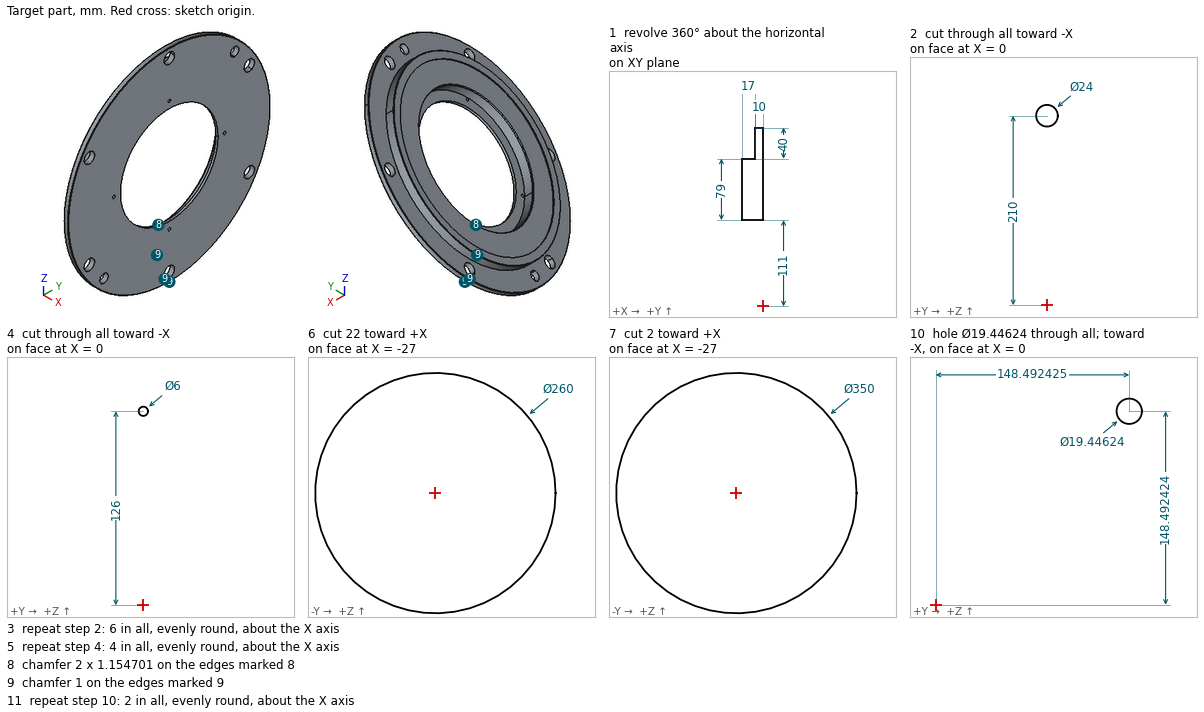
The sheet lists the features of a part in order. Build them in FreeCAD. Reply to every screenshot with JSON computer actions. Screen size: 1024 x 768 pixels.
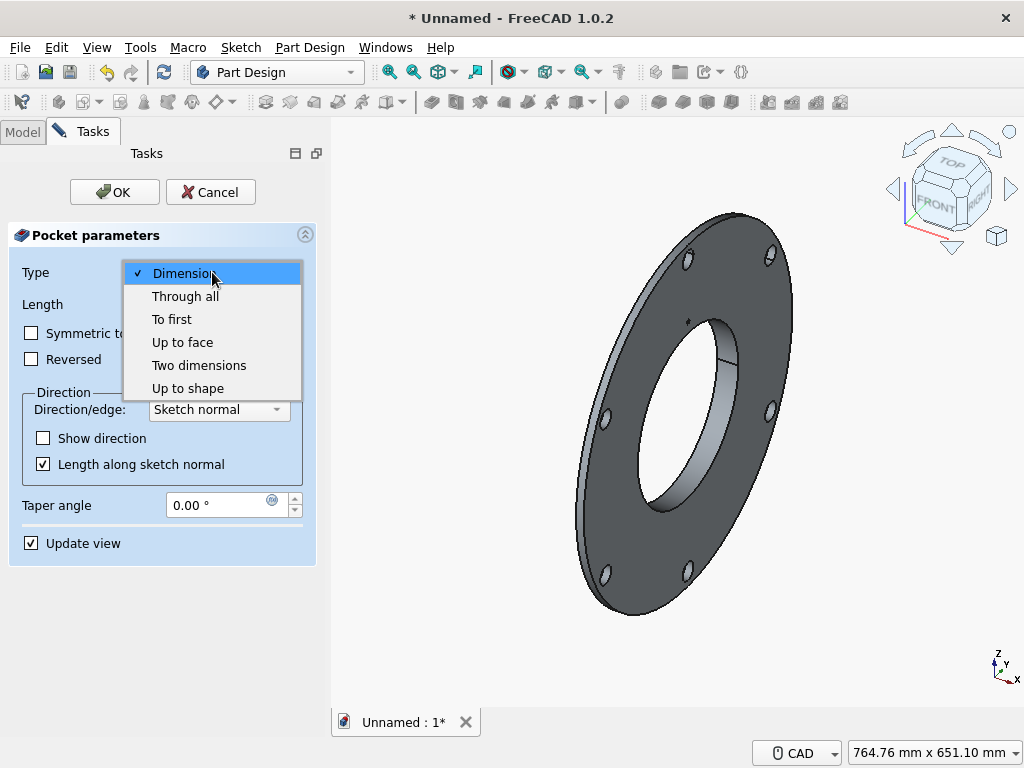
{"action": "left_click", "coordinate": [212, 296]}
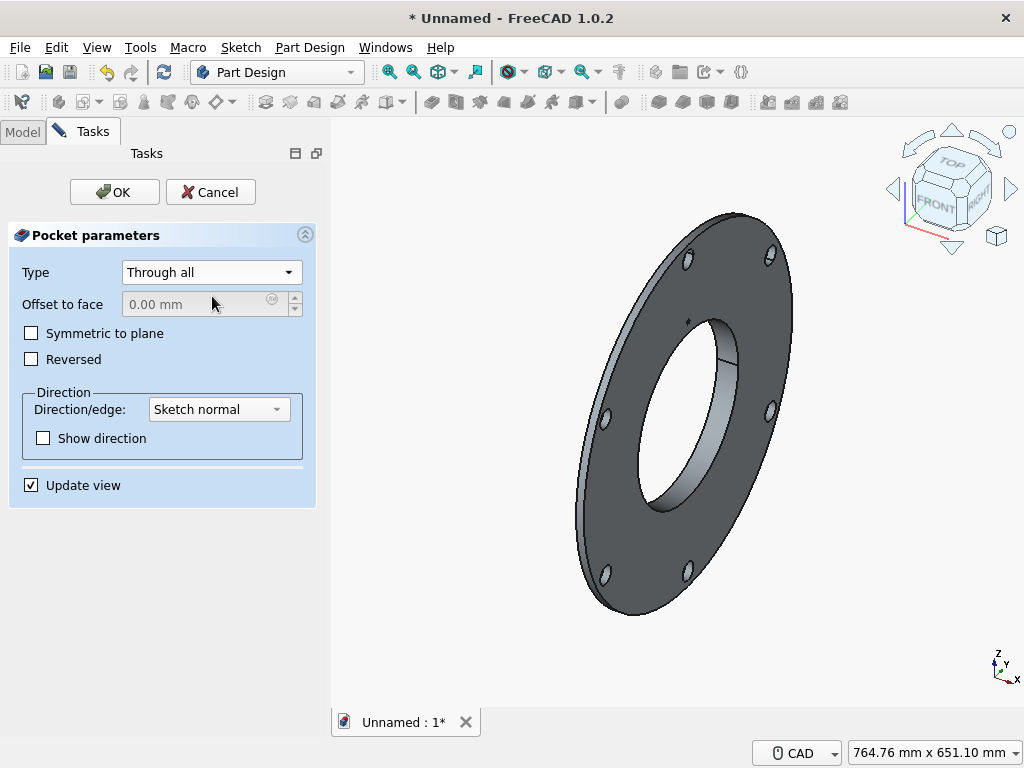
{"action": "left_click", "coordinate": [115, 192]}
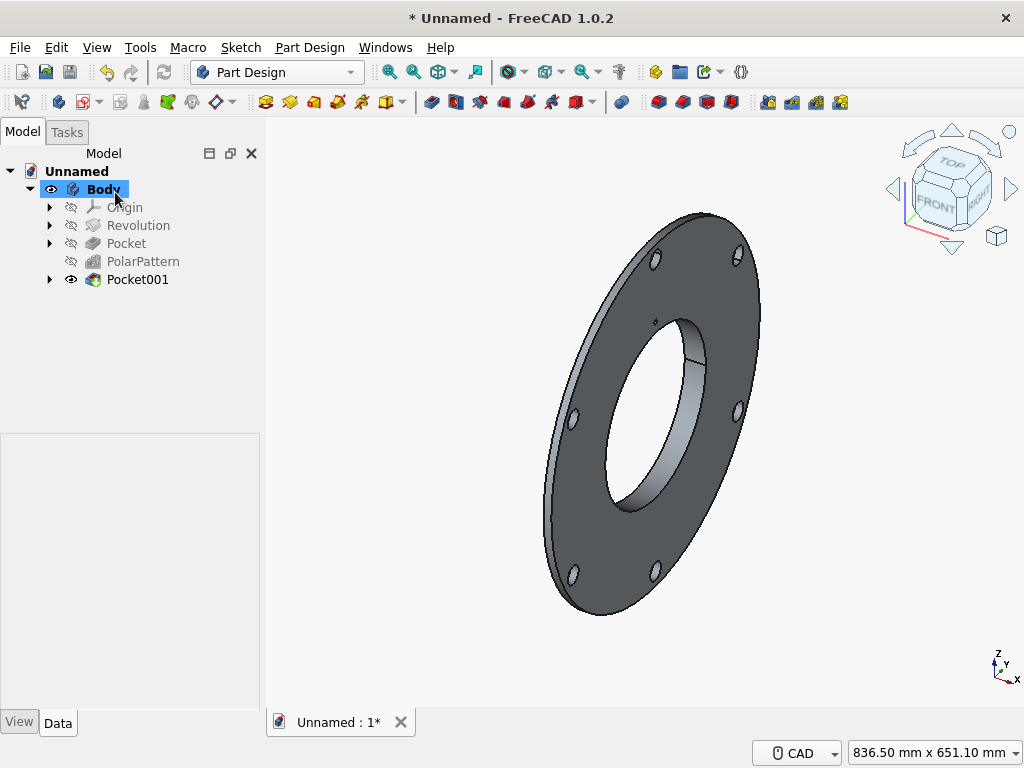
{"action": "left_click", "coordinate": [116, 279]}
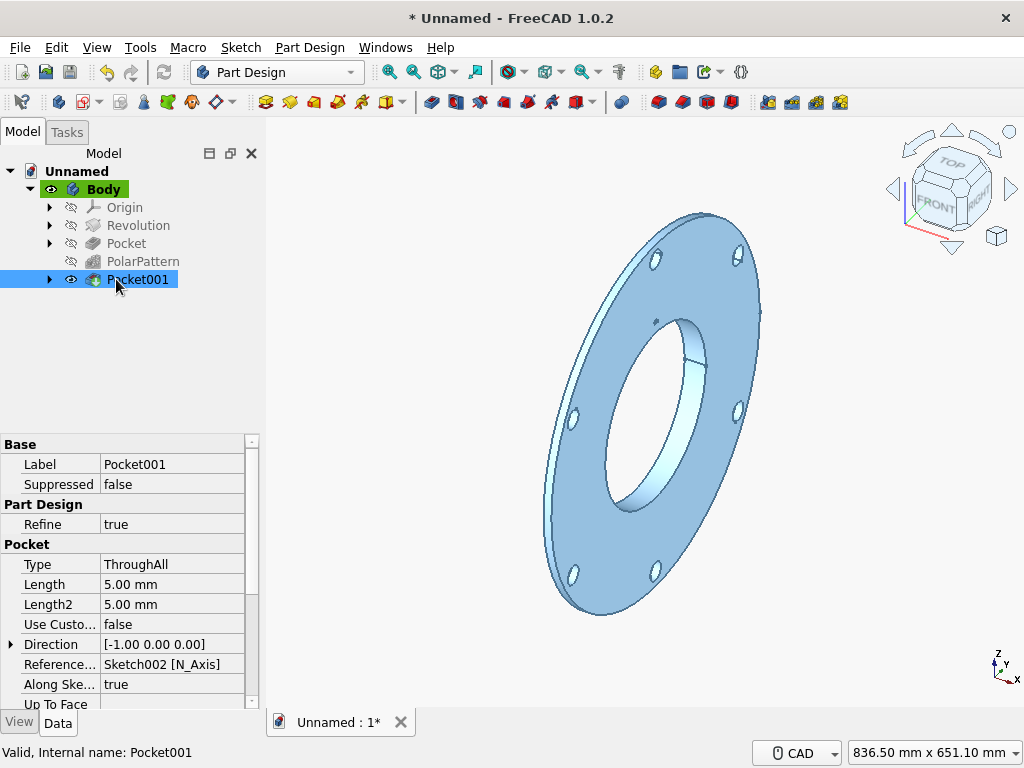
{"action": "left_click", "coordinate": [816, 102]}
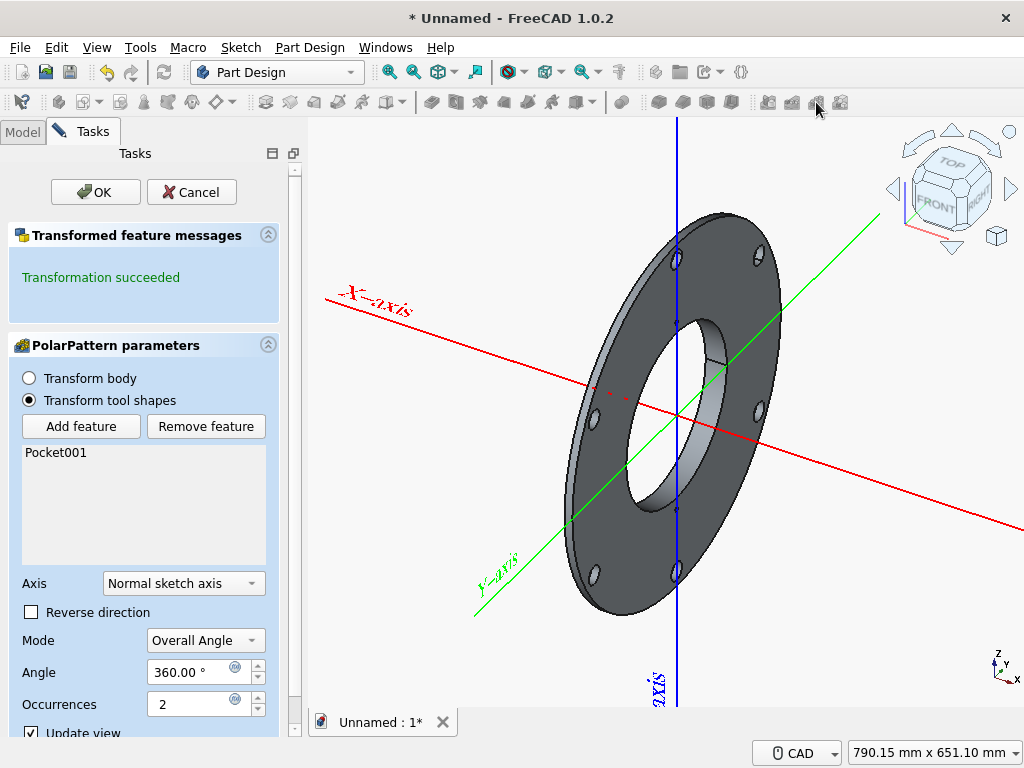
{"action": "left_click", "coordinate": [184, 584]}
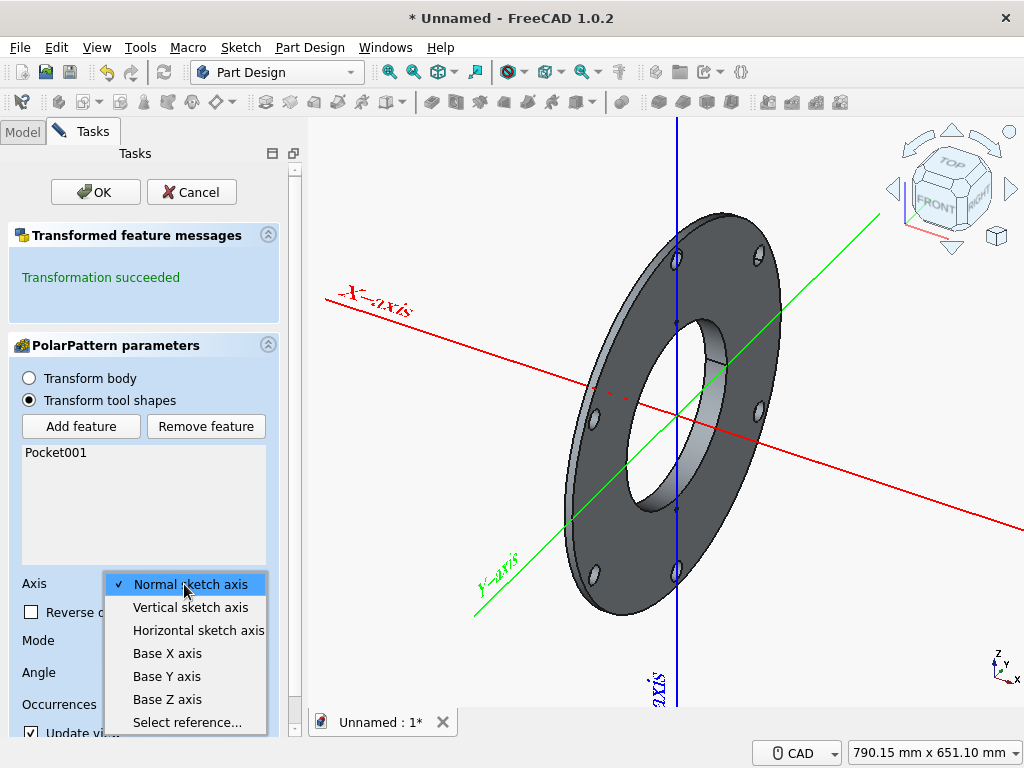
{"action": "left_click", "coordinate": [184, 654]}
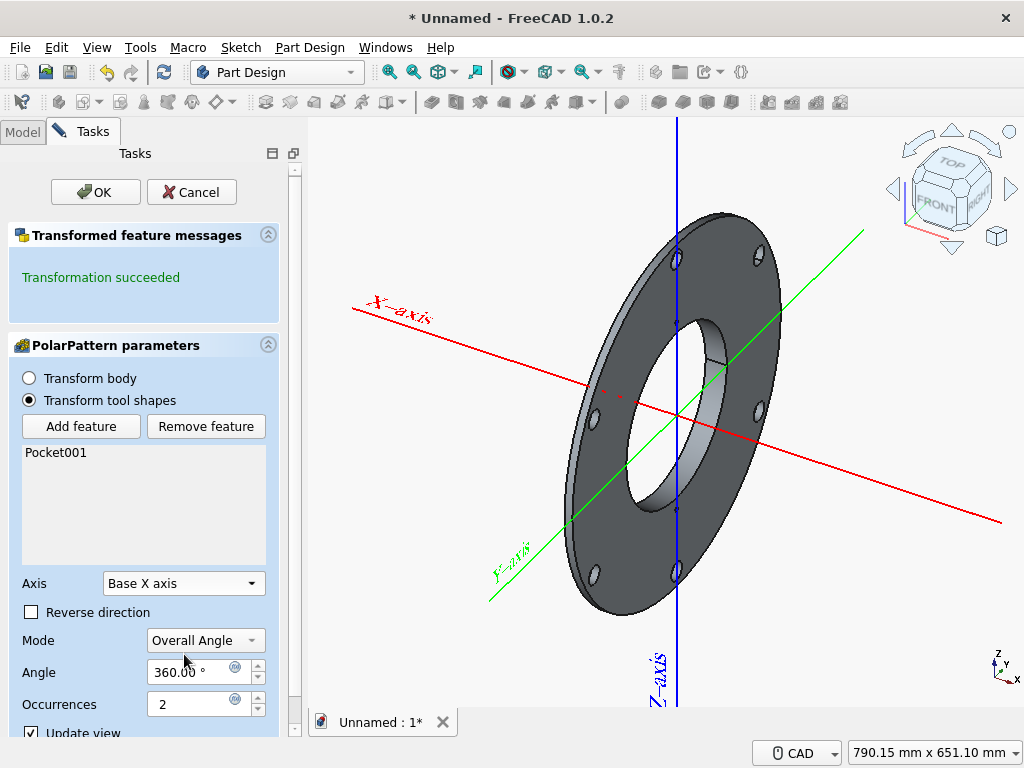
{"action": "triple_click", "coordinate": [198, 704]}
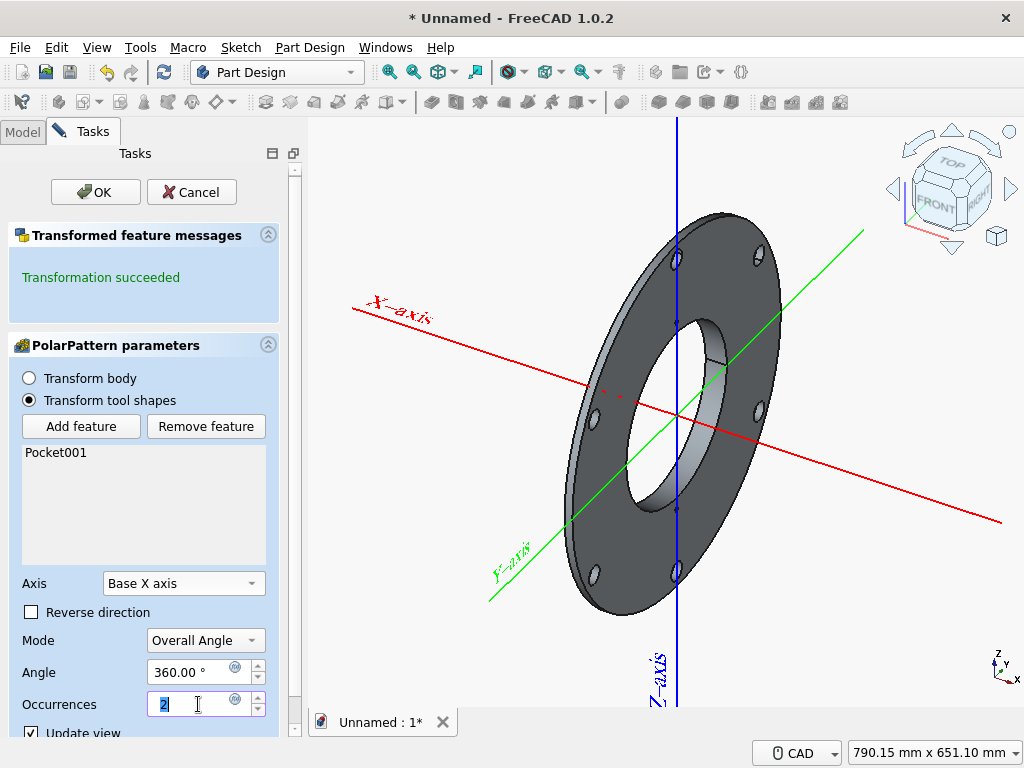
{"action": "type", "text": "4"}
{"action": "key", "text": "Tab"}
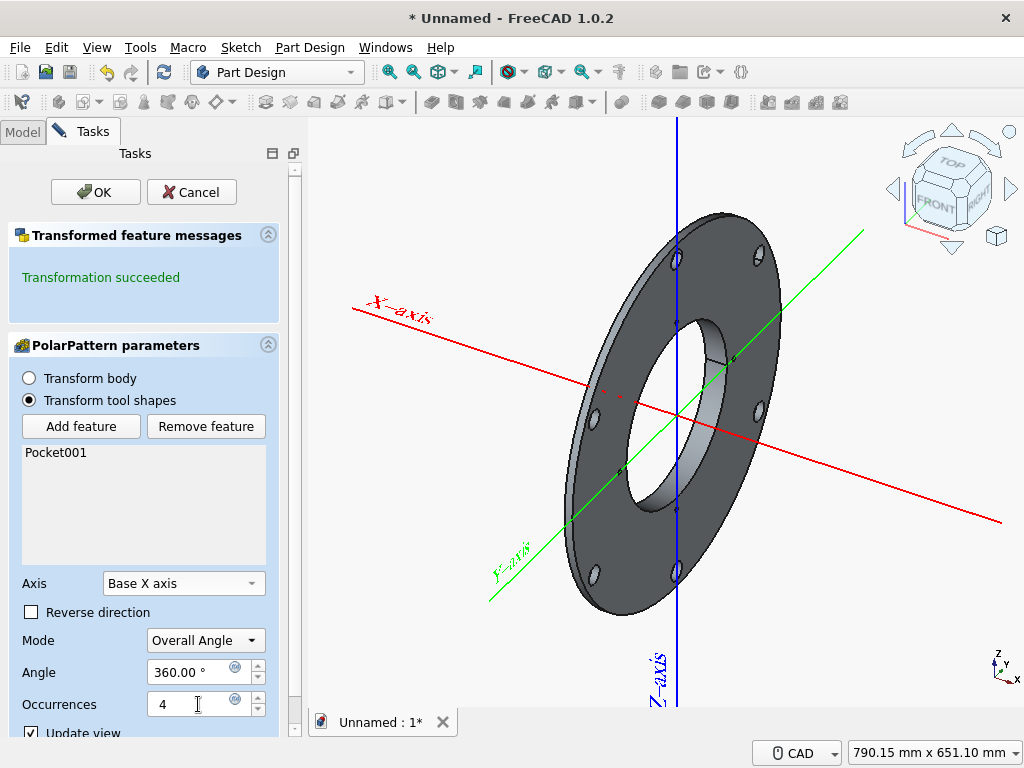
{"action": "left_click", "coordinate": [96, 192]}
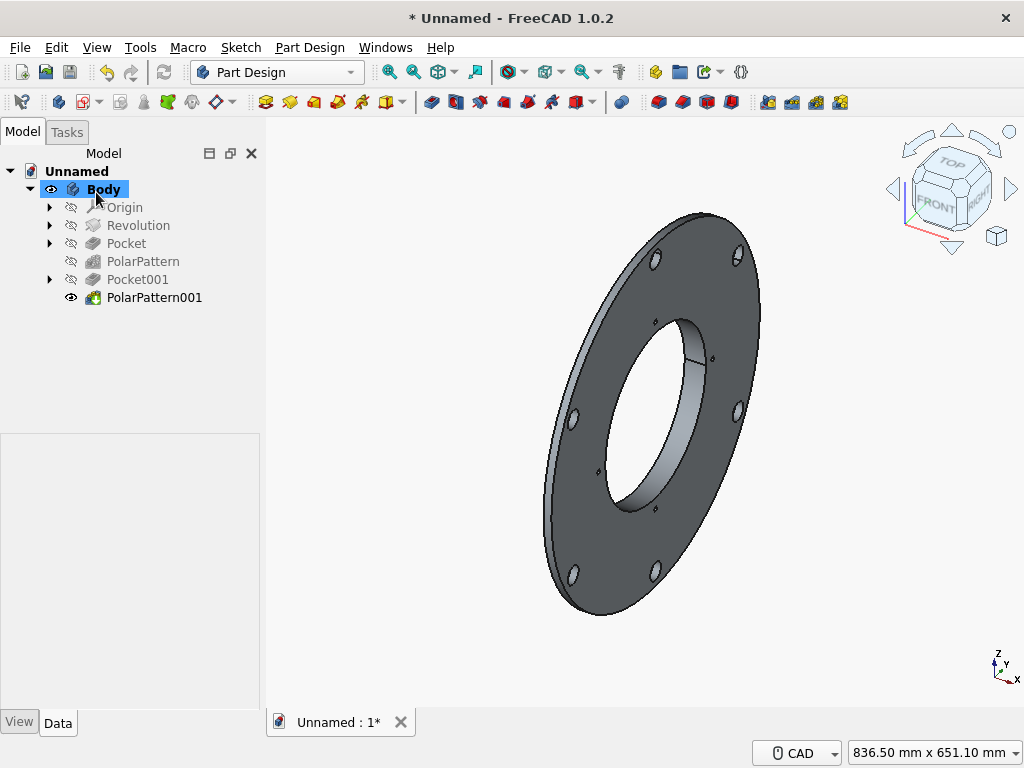
{"action": "key", "text": "6"}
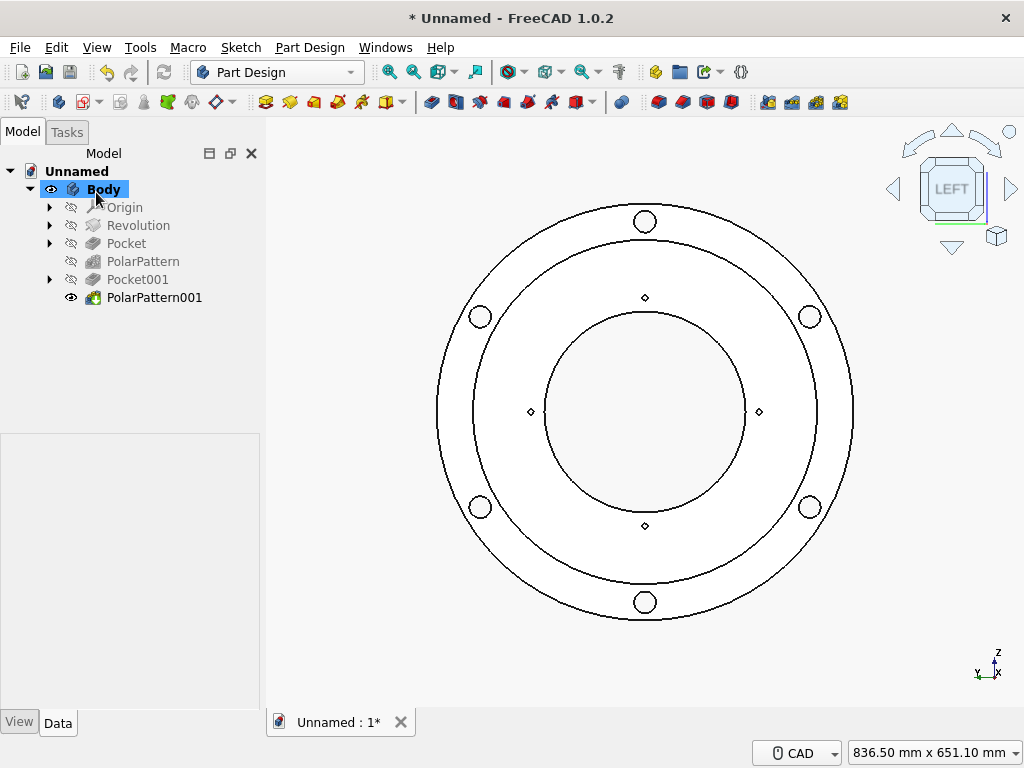
{"action": "left_click", "coordinate": [547, 509]}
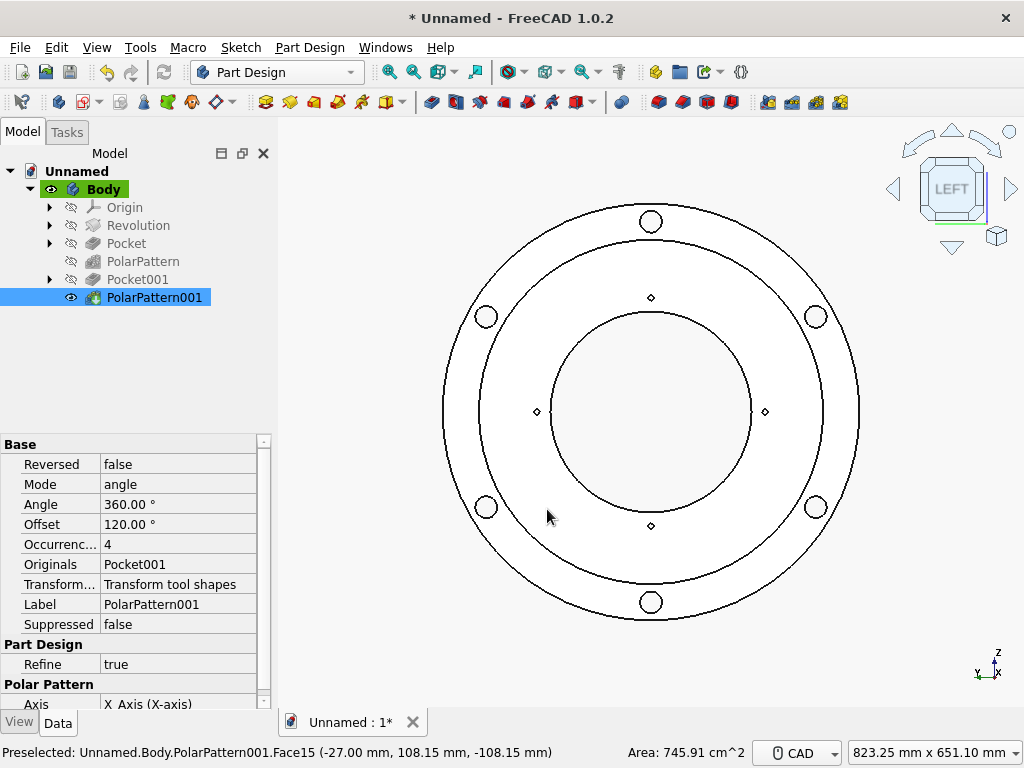
{"action": "left_click", "coordinate": [84, 102]}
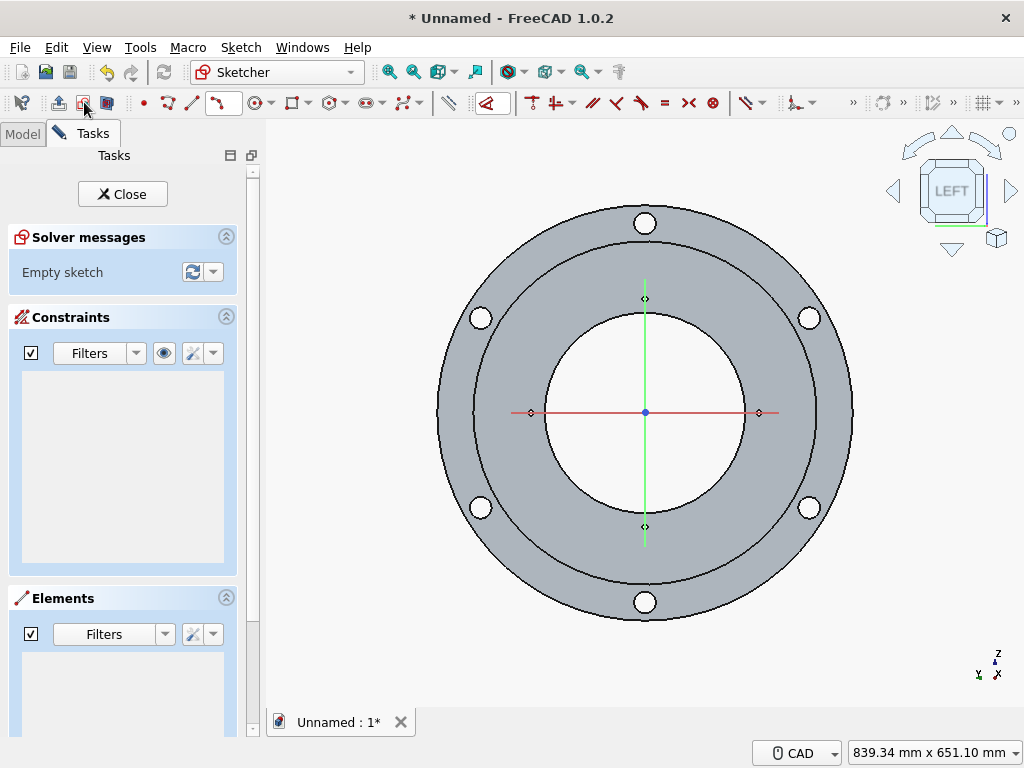
{"action": "scroll", "coordinate": [784, 413], "scroll_direction": "up", "scroll_amount": 2}